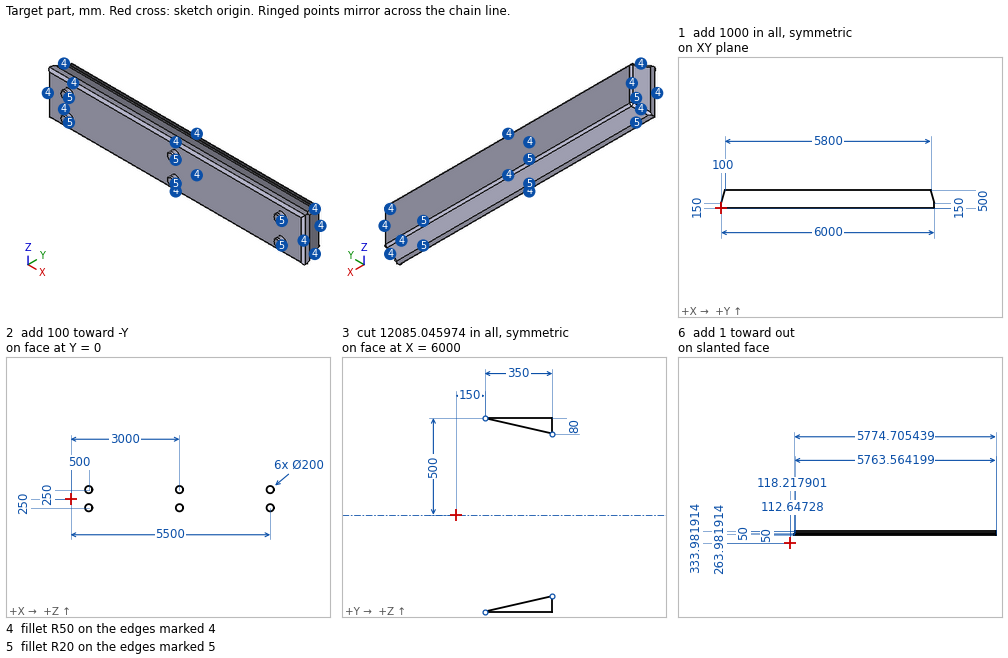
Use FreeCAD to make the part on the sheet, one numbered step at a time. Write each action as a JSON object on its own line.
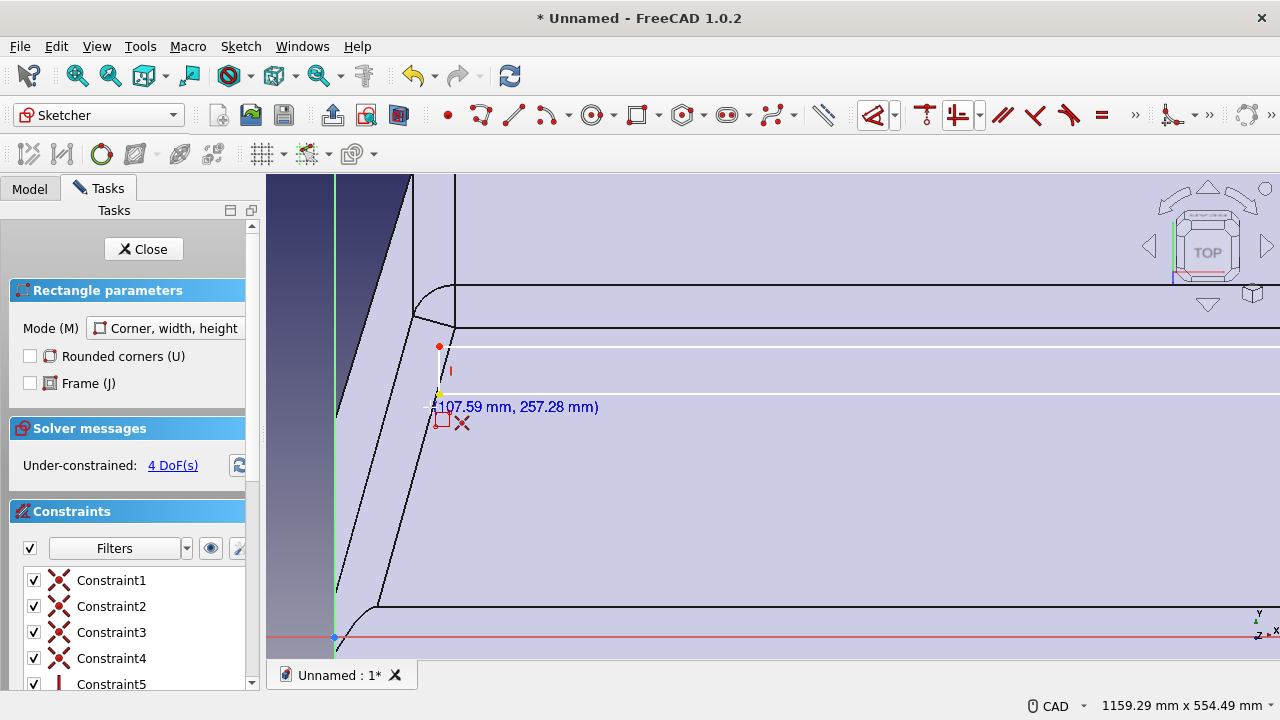
{"action": "left_click", "coordinate": [433, 406]}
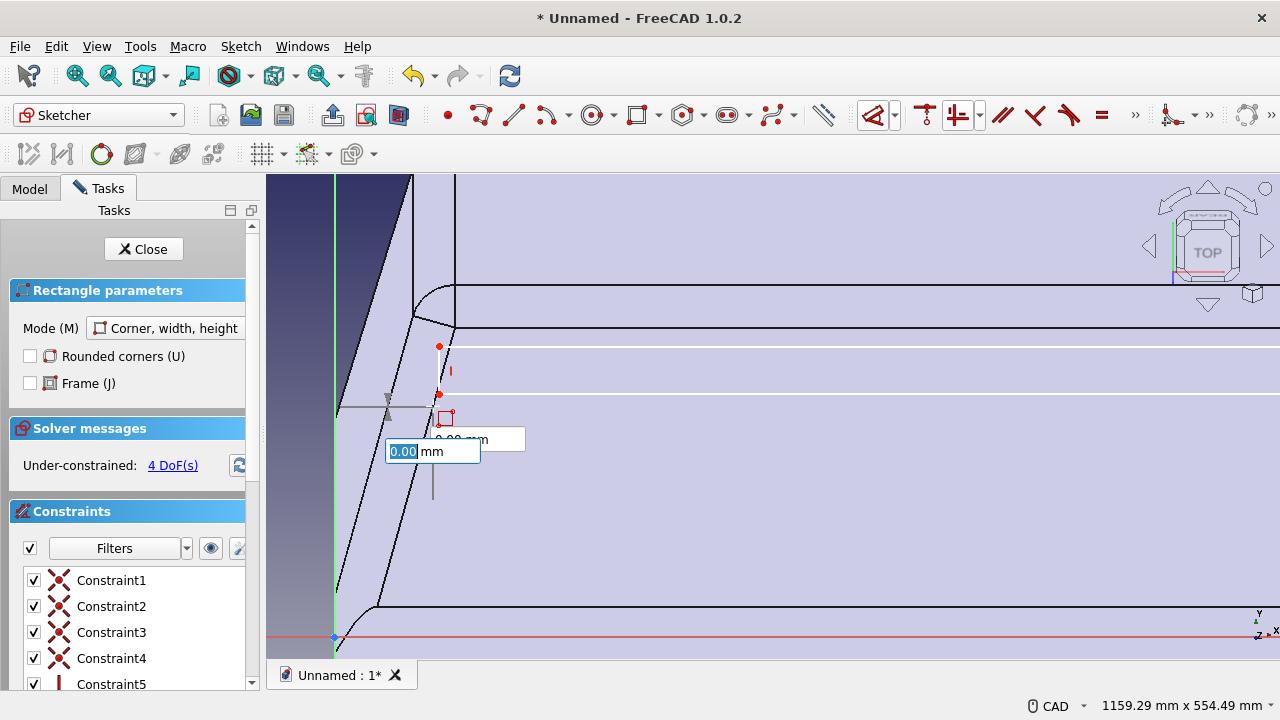
{"action": "scroll", "coordinate": [430, 407], "scroll_direction": "down", "scroll_amount": 11}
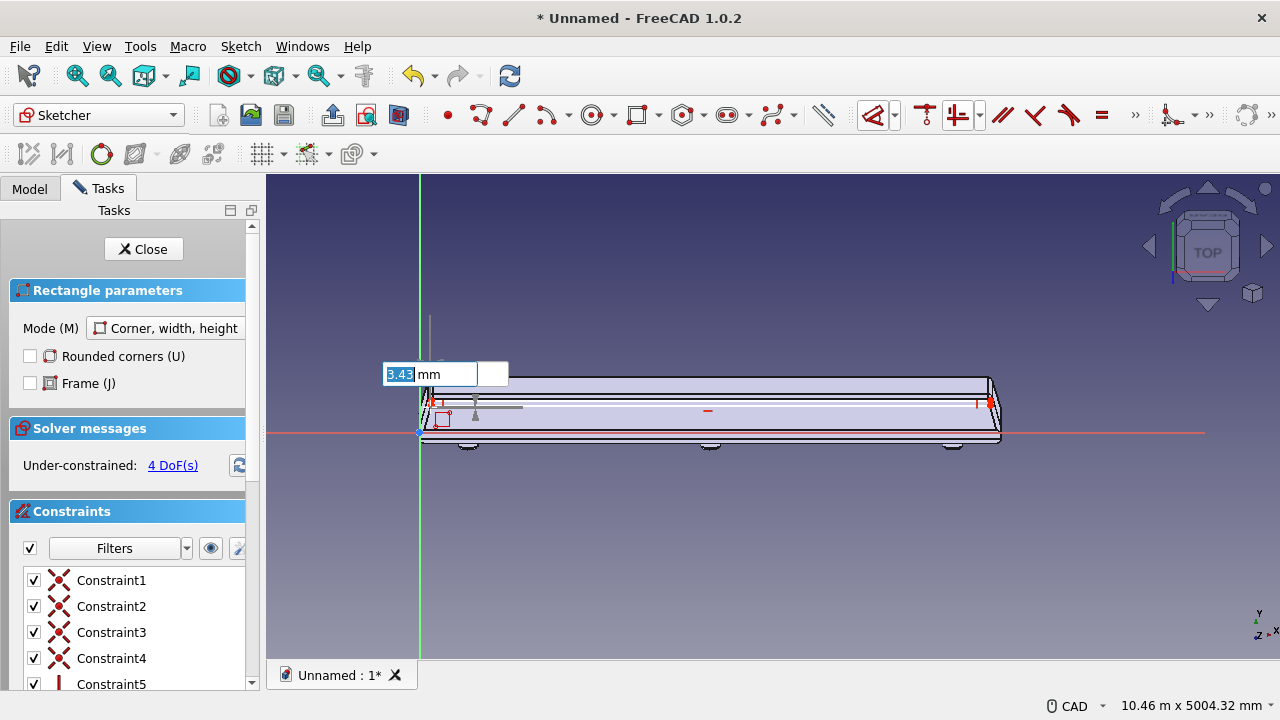
{"action": "scroll", "coordinate": [990, 412], "scroll_direction": "up", "scroll_amount": 5}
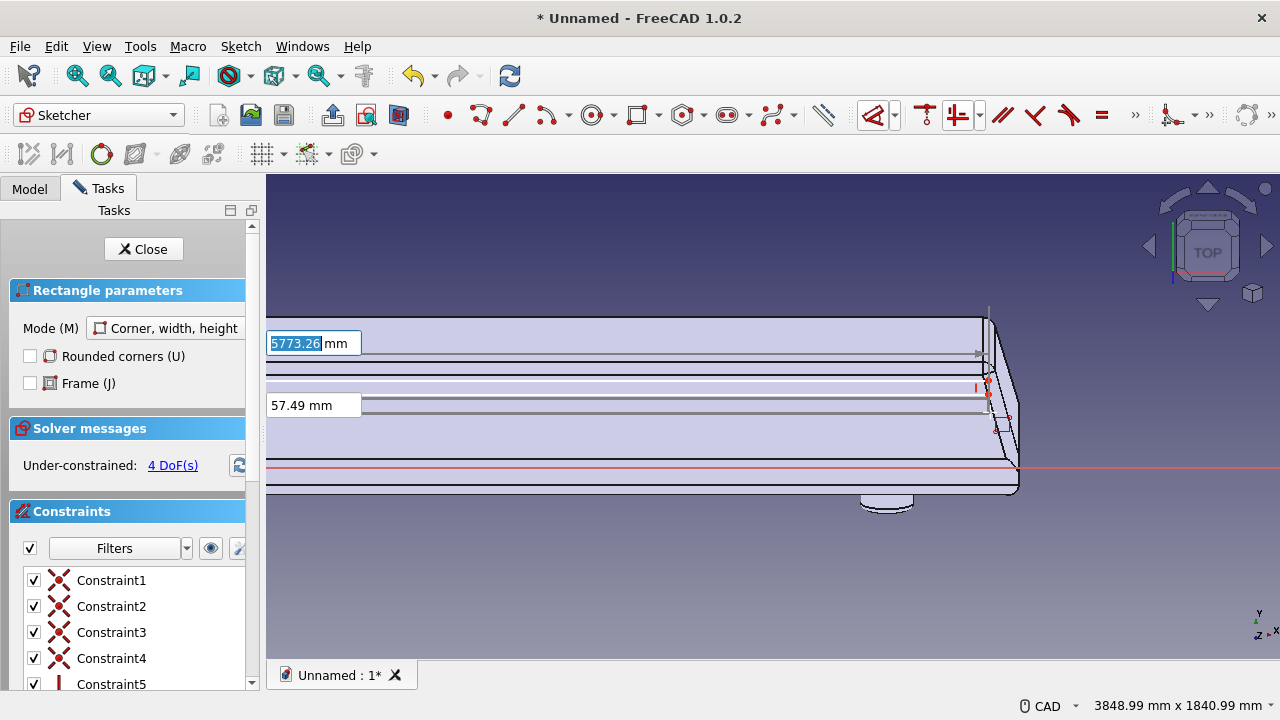
{"action": "left_click", "coordinate": [989, 412]}
{"action": "key", "text": "Escape"}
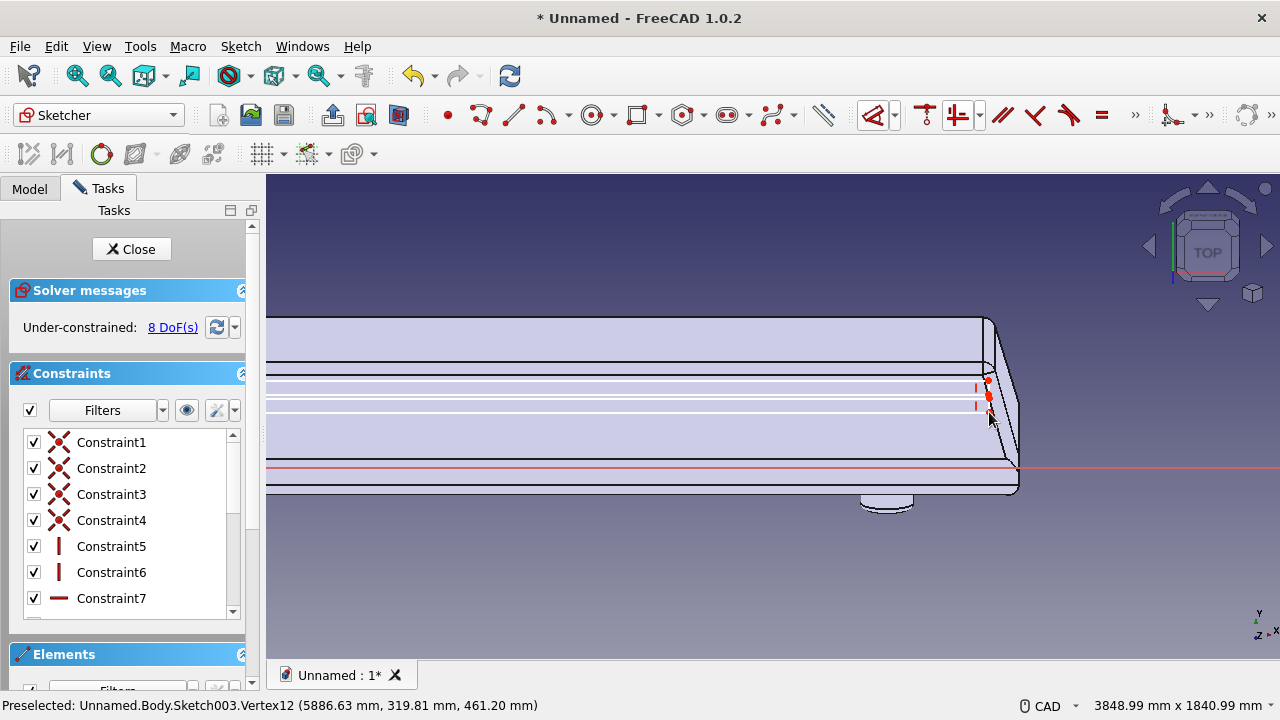
{"action": "scroll", "coordinate": [990, 412], "scroll_direction": "down", "scroll_amount": 5}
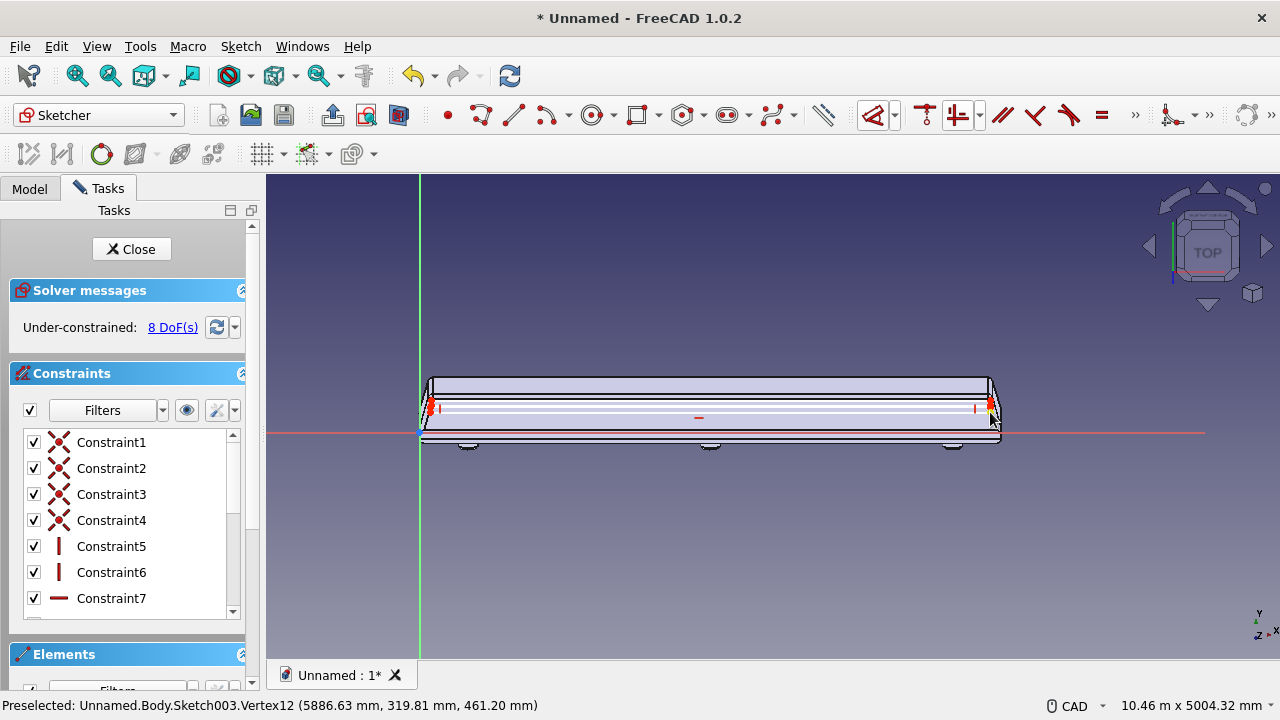
{"action": "scroll", "coordinate": [431, 403], "scroll_direction": "up", "scroll_amount": 11}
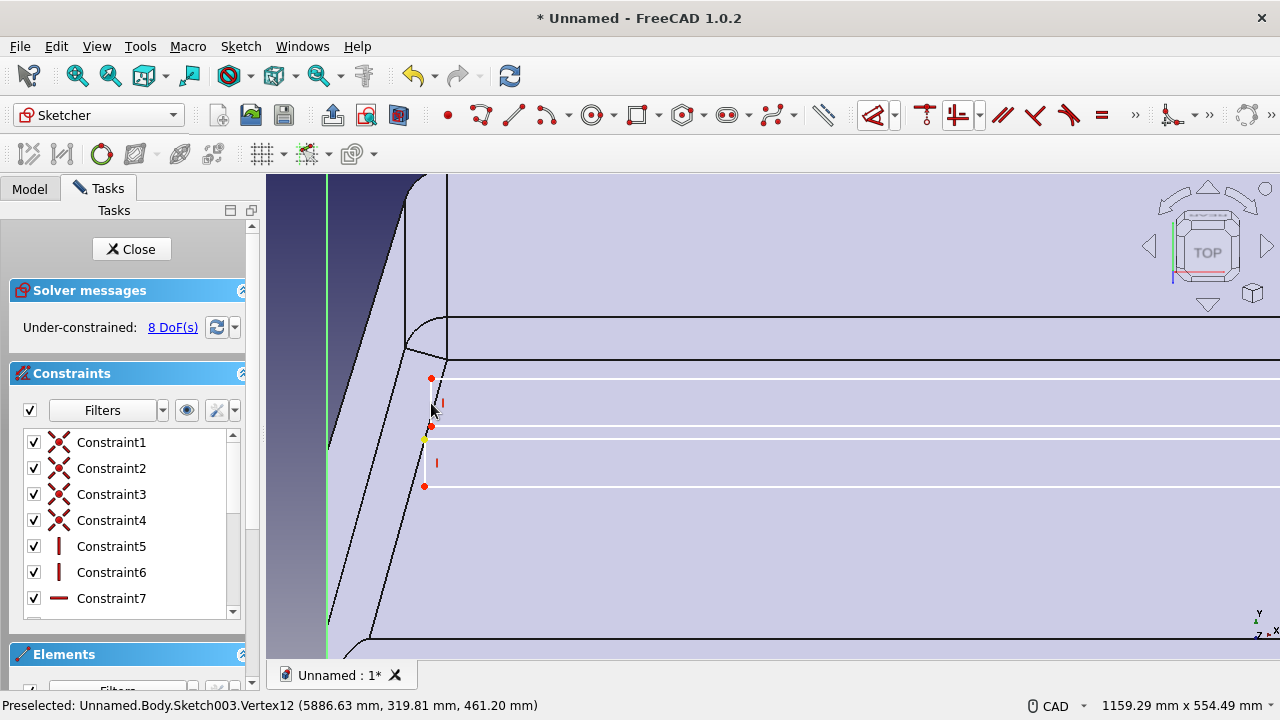
{"action": "left_click", "coordinate": [431, 403]}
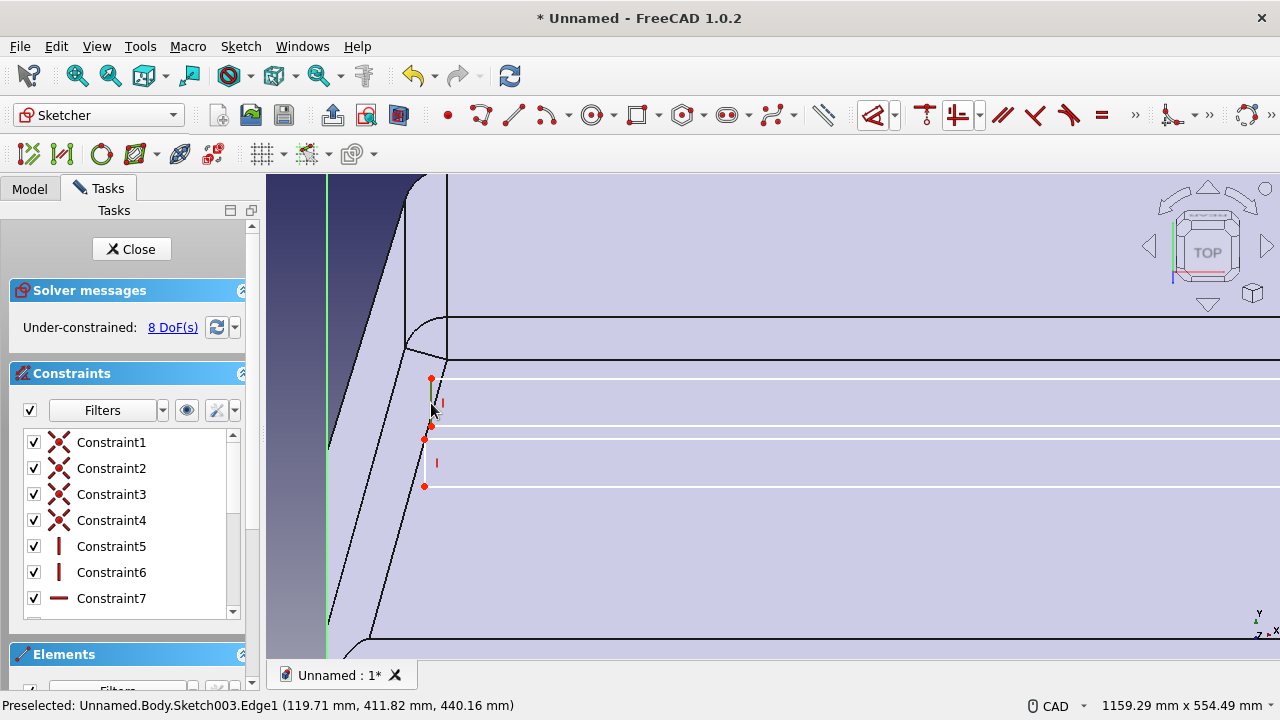
{"action": "left_click", "coordinate": [894, 116]}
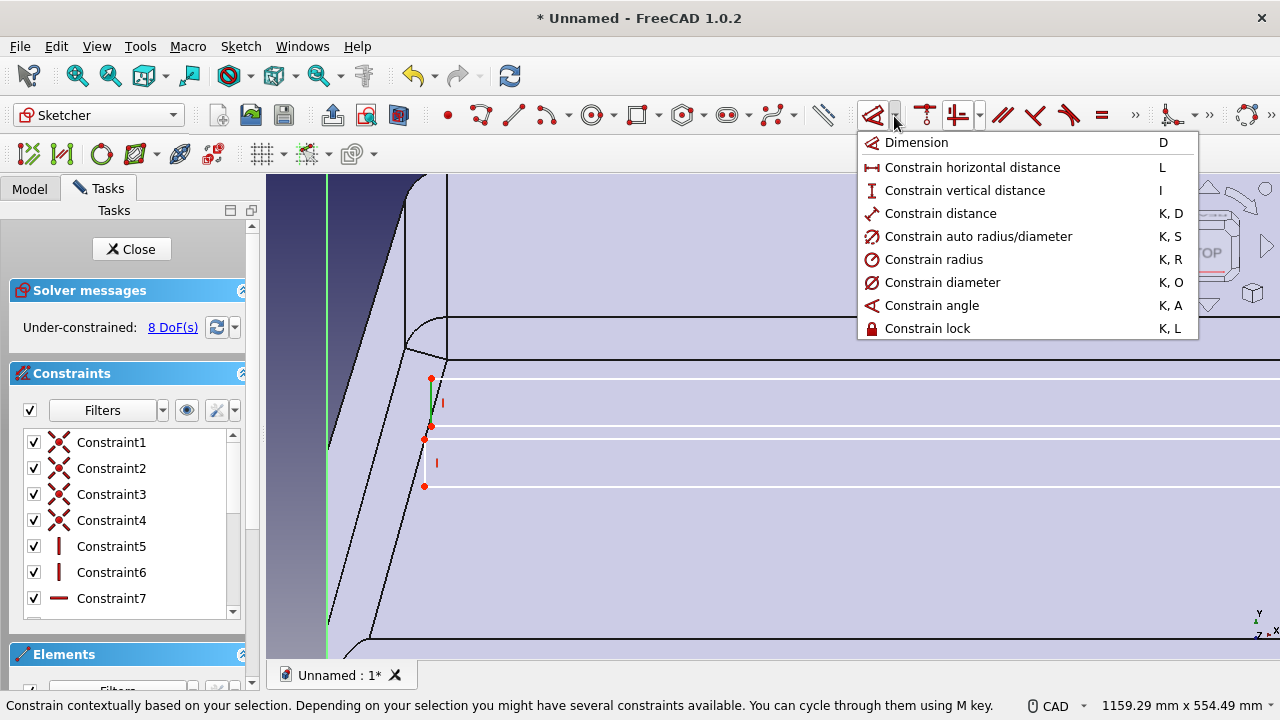
{"action": "left_click", "coordinate": [1028, 190]}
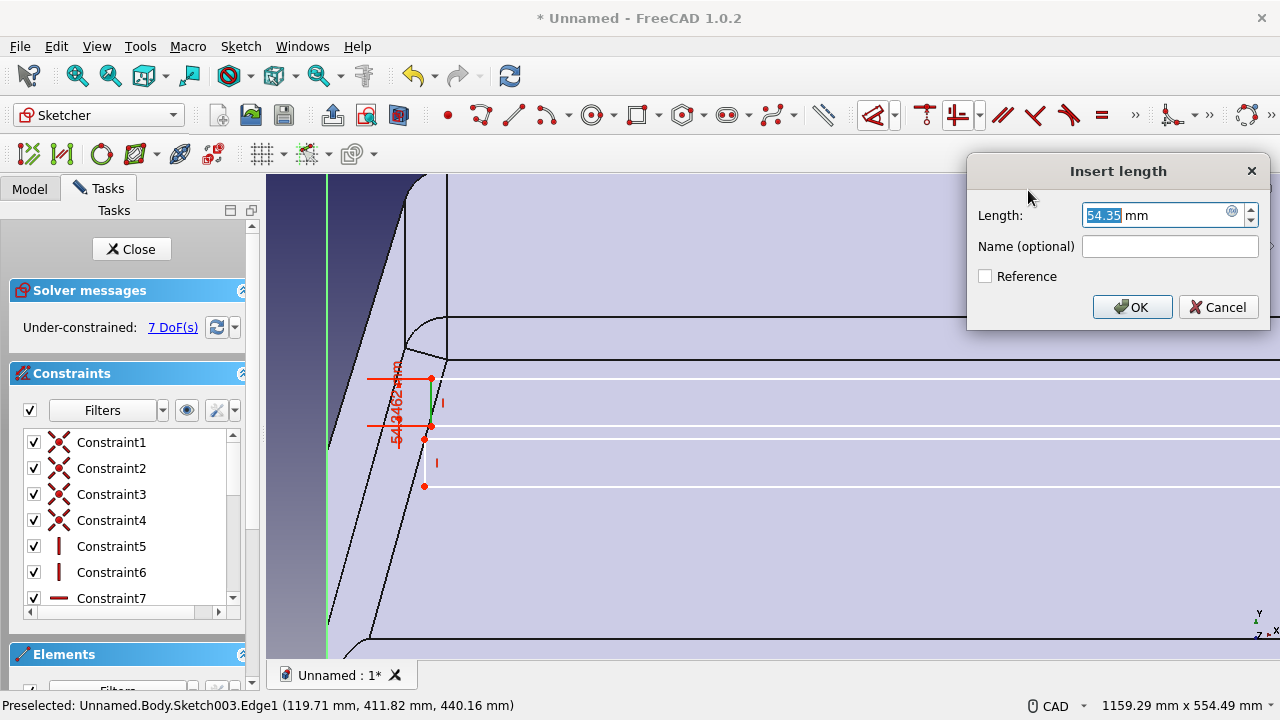
{"action": "type", "text": "50"}
{"action": "key", "text": "Return"}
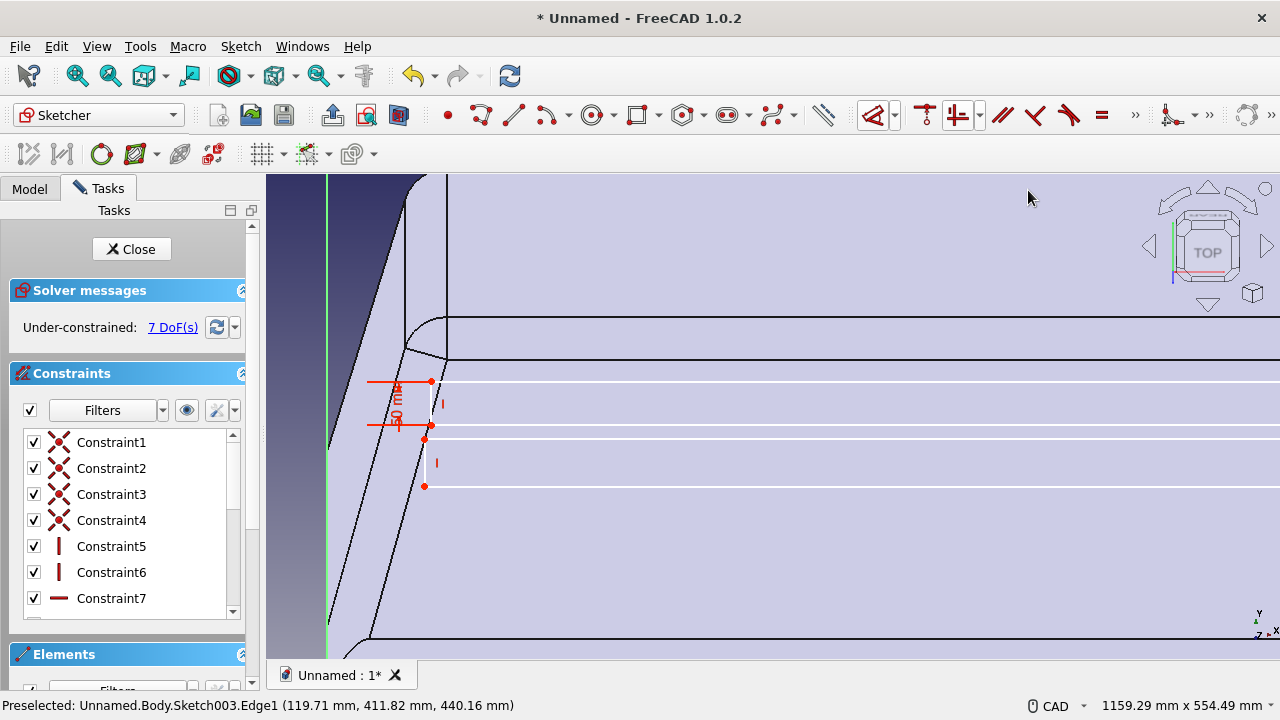
{"action": "left_click", "coordinate": [425, 453]}